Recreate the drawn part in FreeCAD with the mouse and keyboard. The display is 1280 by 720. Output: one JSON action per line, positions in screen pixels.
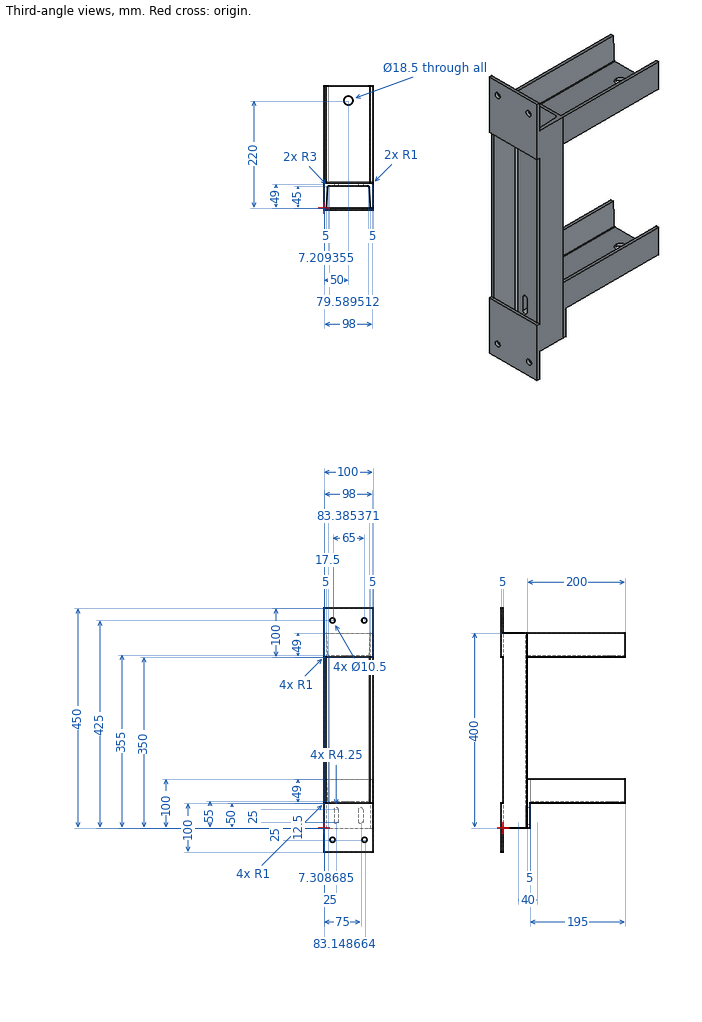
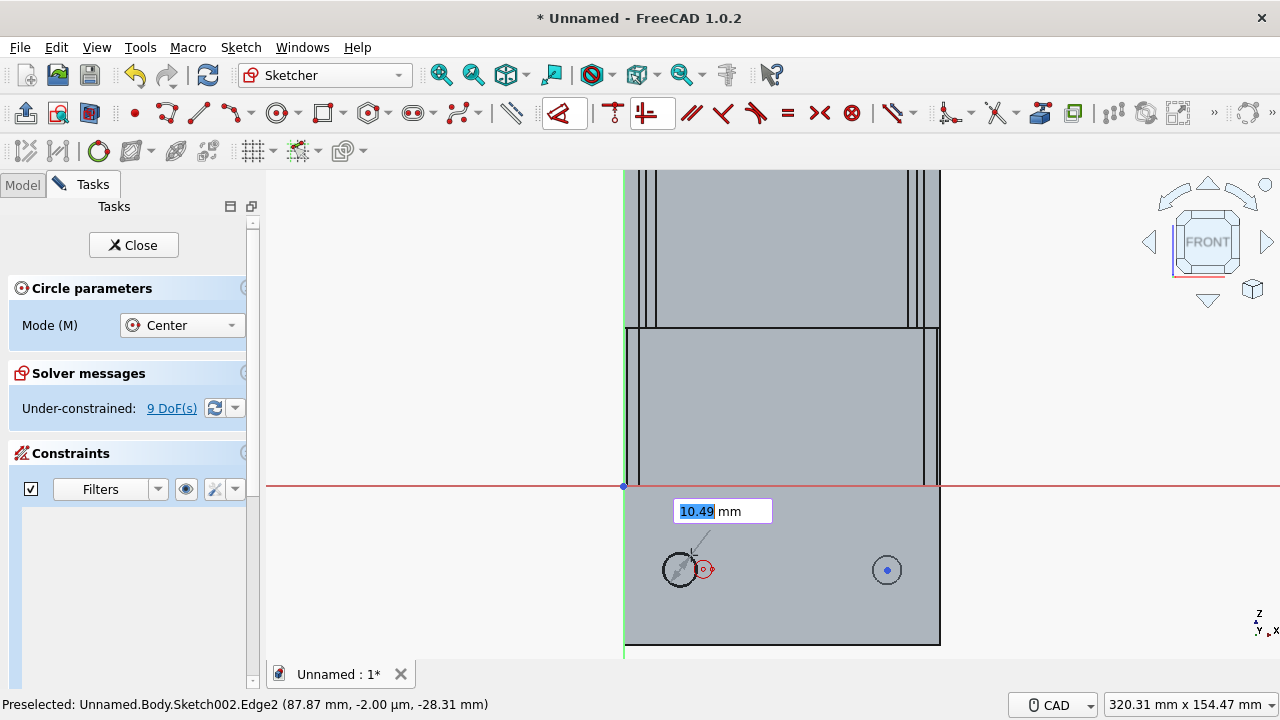
{"action": "left_click", "coordinate": [691, 554]}
{"action": "key", "text": "Escape"}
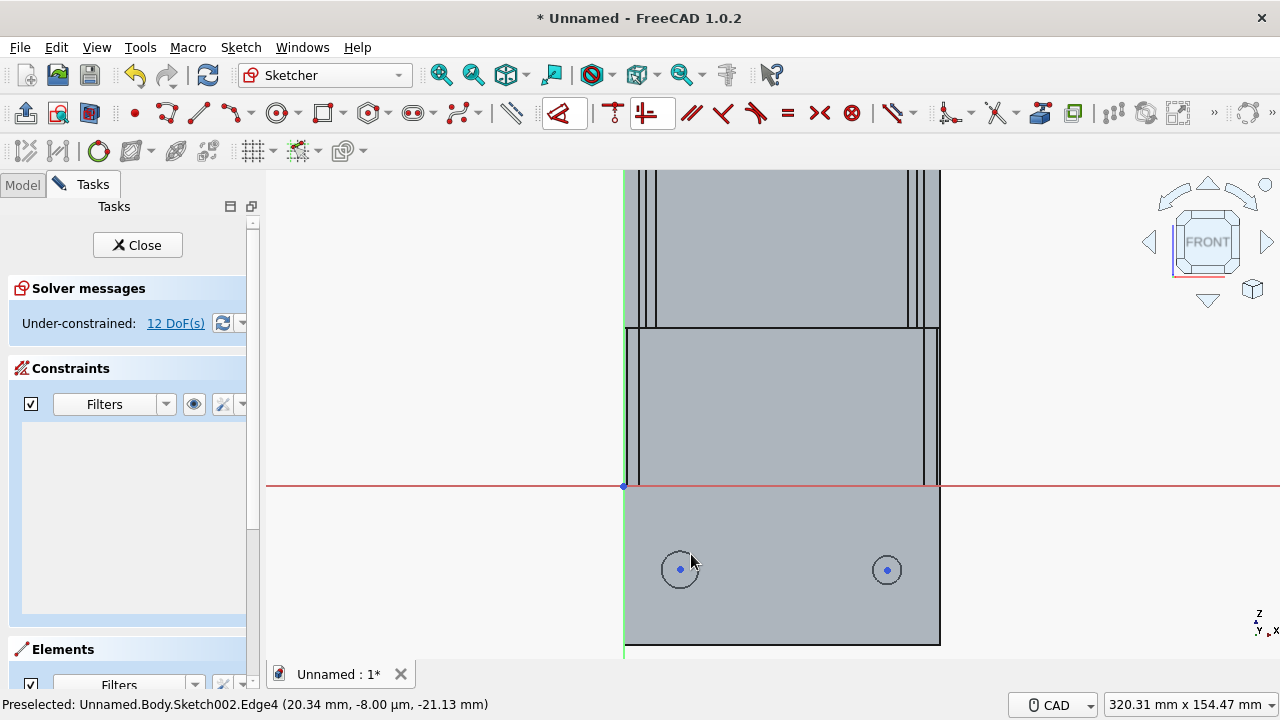
{"action": "scroll", "coordinate": [690, 557], "scroll_direction": "down", "scroll_amount": 8}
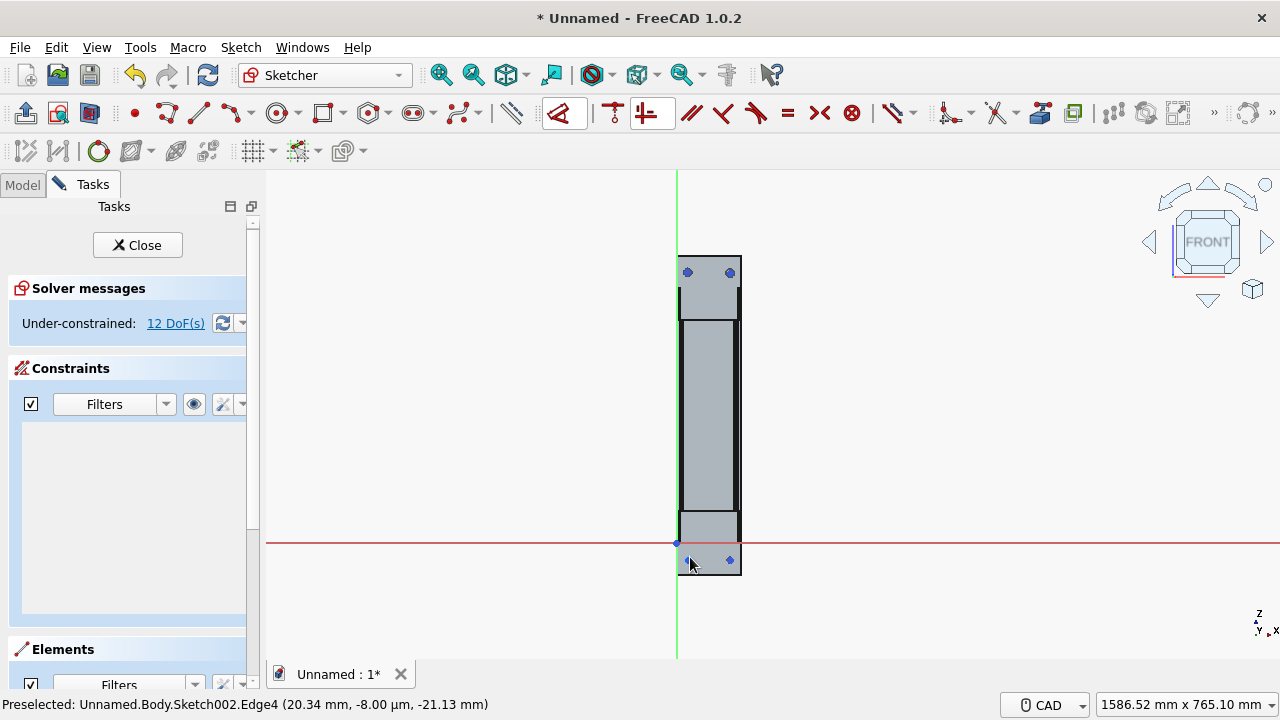
{"action": "scroll", "coordinate": [691, 270], "scroll_direction": "up", "scroll_amount": 7}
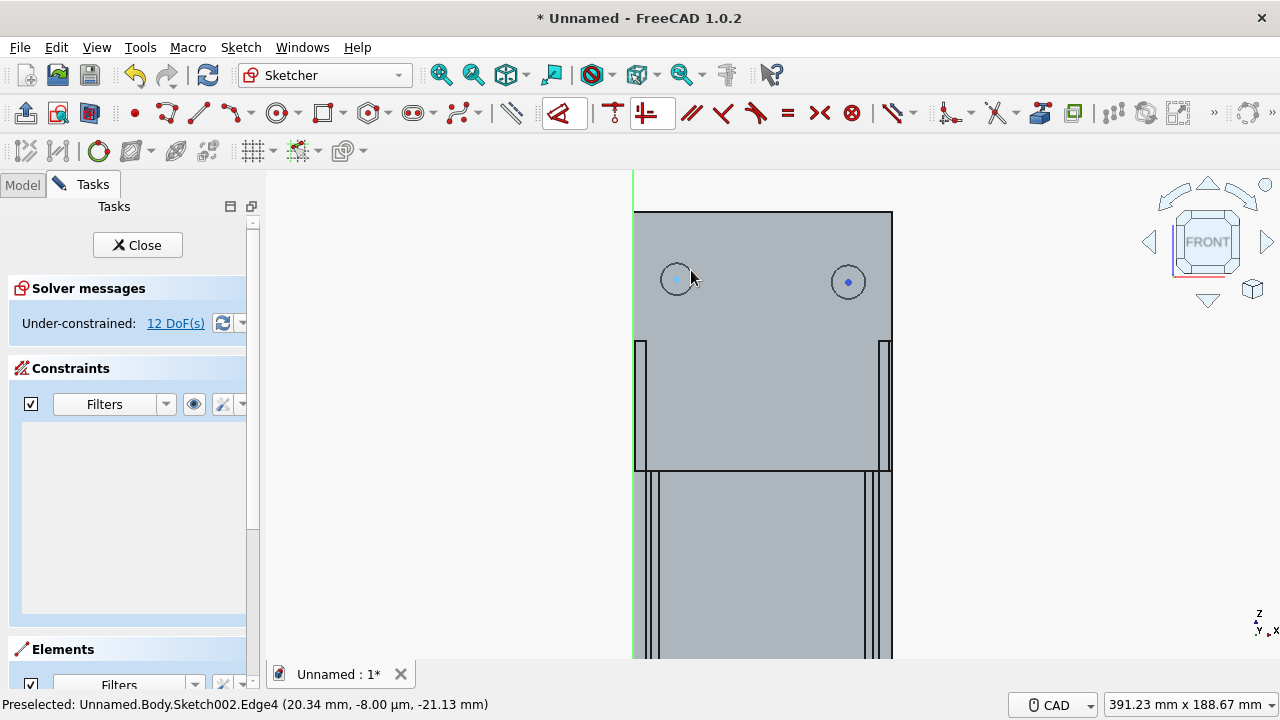
{"action": "left_click", "coordinate": [688, 268]}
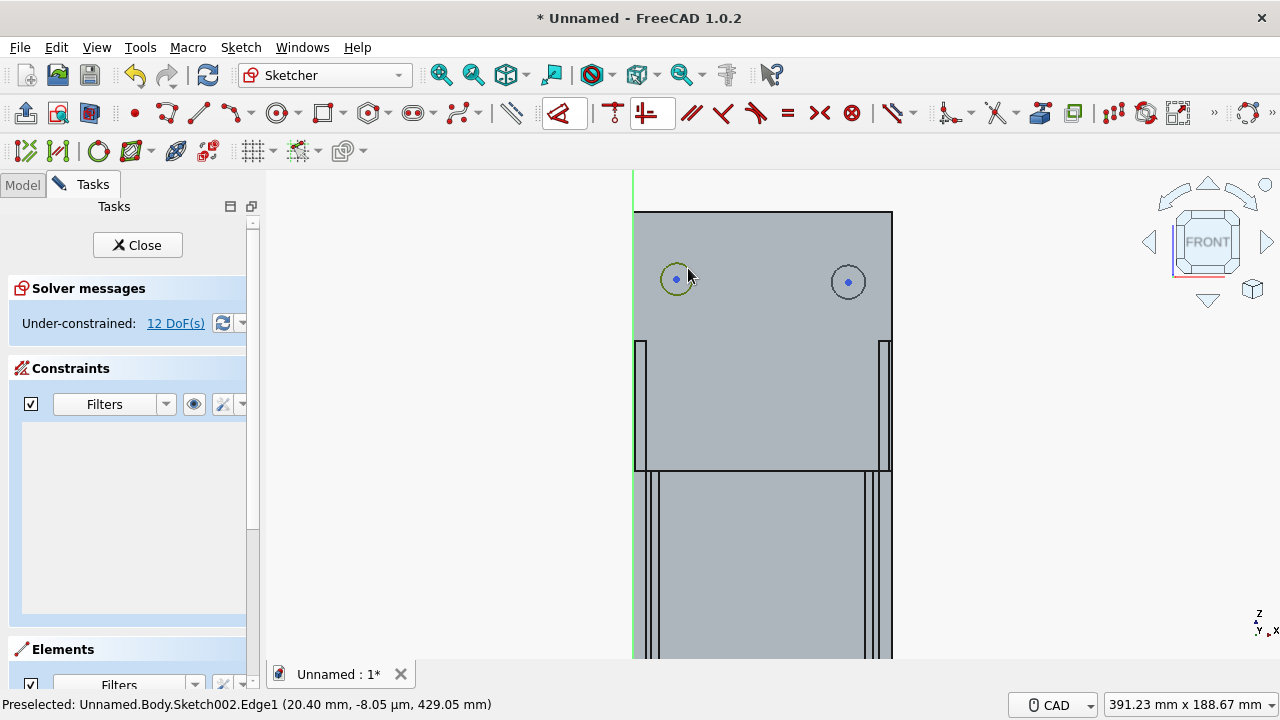
{"action": "left_click", "coordinate": [860, 270]}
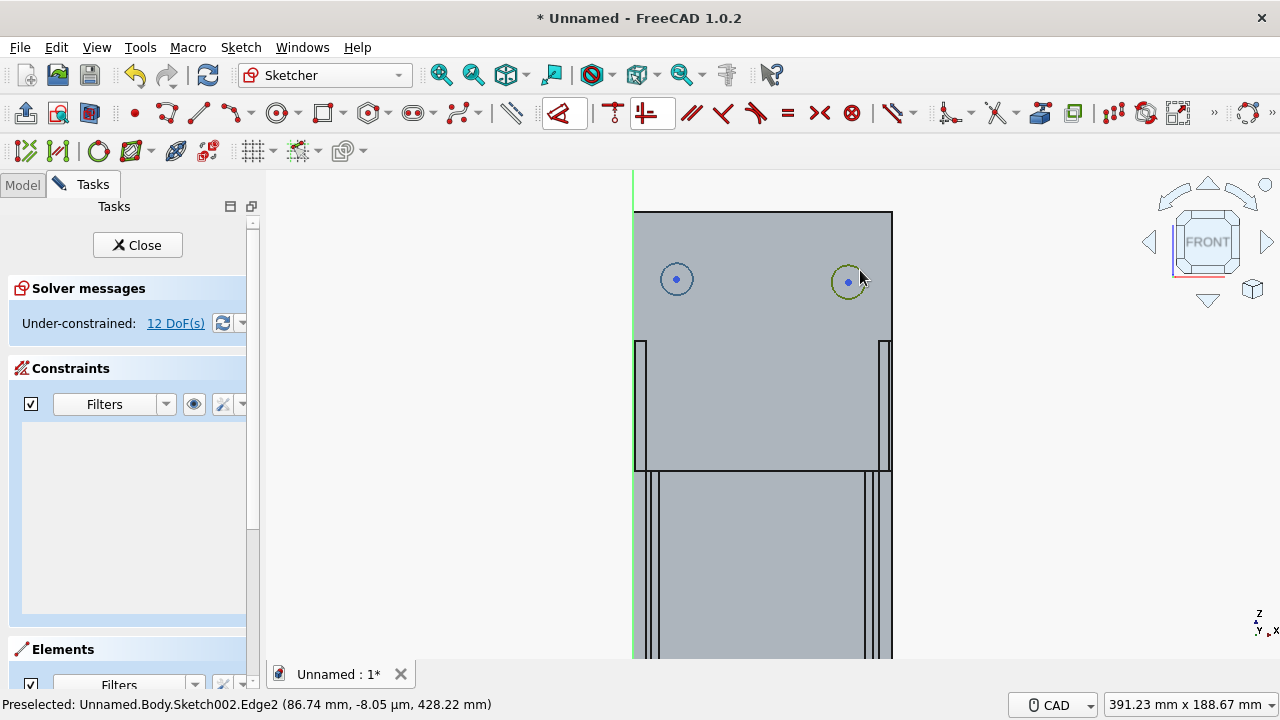
{"action": "scroll", "coordinate": [691, 269], "scroll_direction": "down", "scroll_amount": 7}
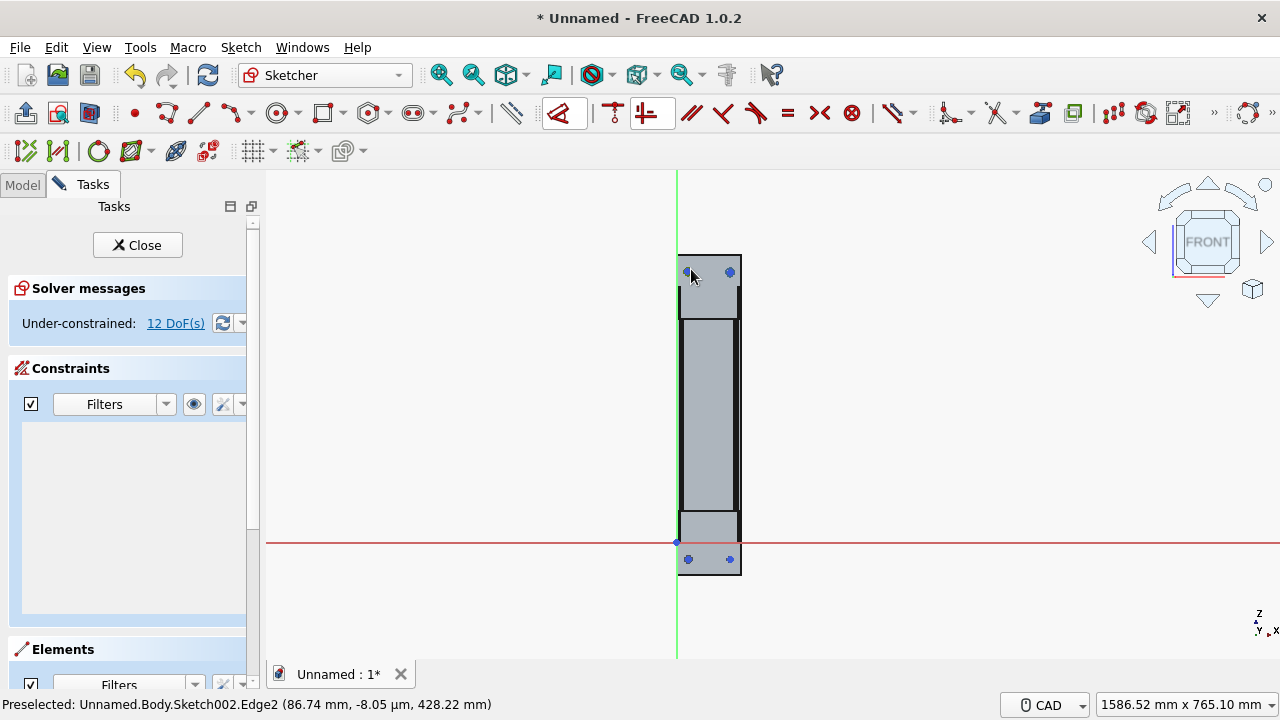
{"action": "scroll", "coordinate": [732, 557], "scroll_direction": "up", "scroll_amount": 8}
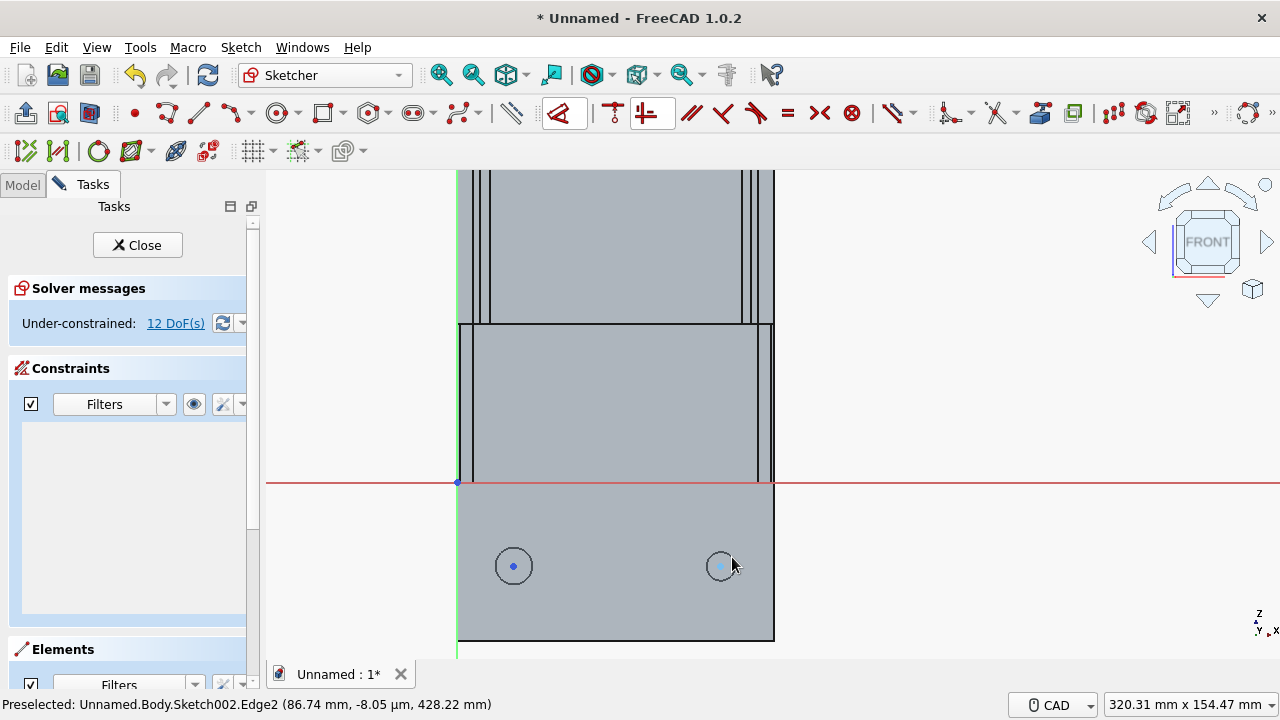
{"action": "left_click", "coordinate": [731, 556]}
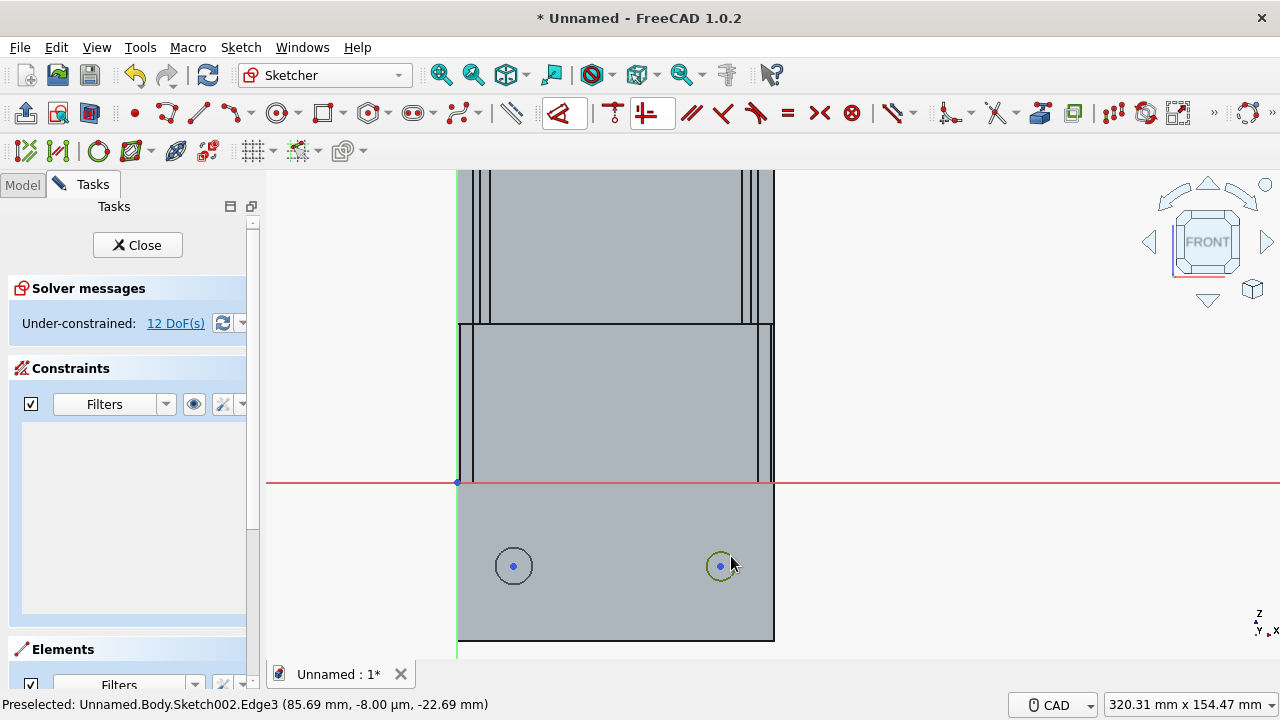
{"action": "left_click", "coordinate": [527, 553]}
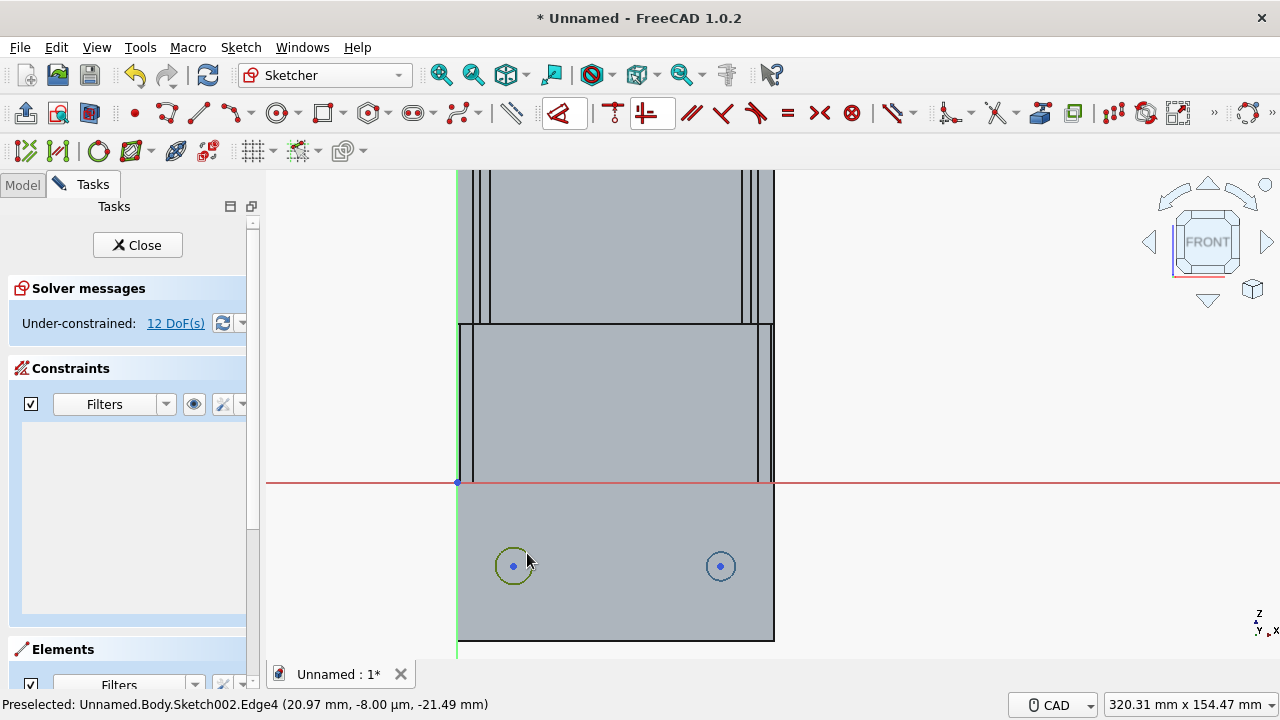
{"action": "left_click", "coordinate": [788, 114]}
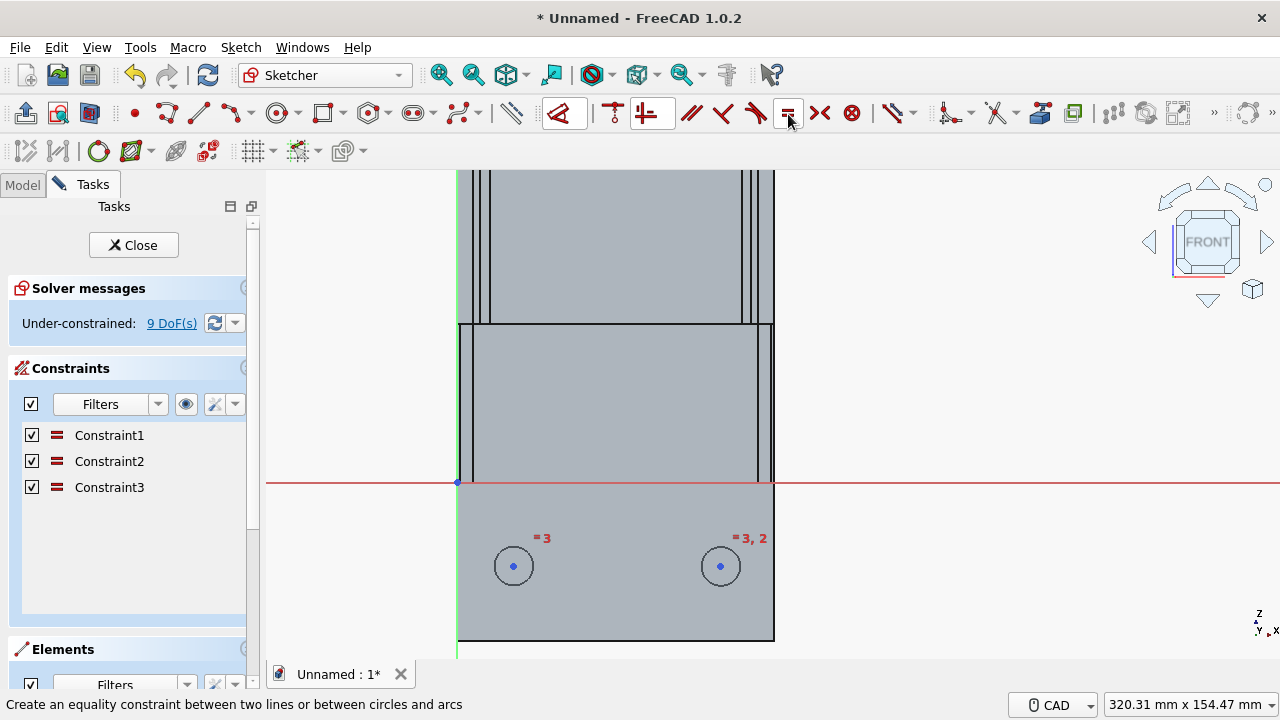
{"action": "scroll", "coordinate": [732, 557], "scroll_direction": "down", "scroll_amount": 8}